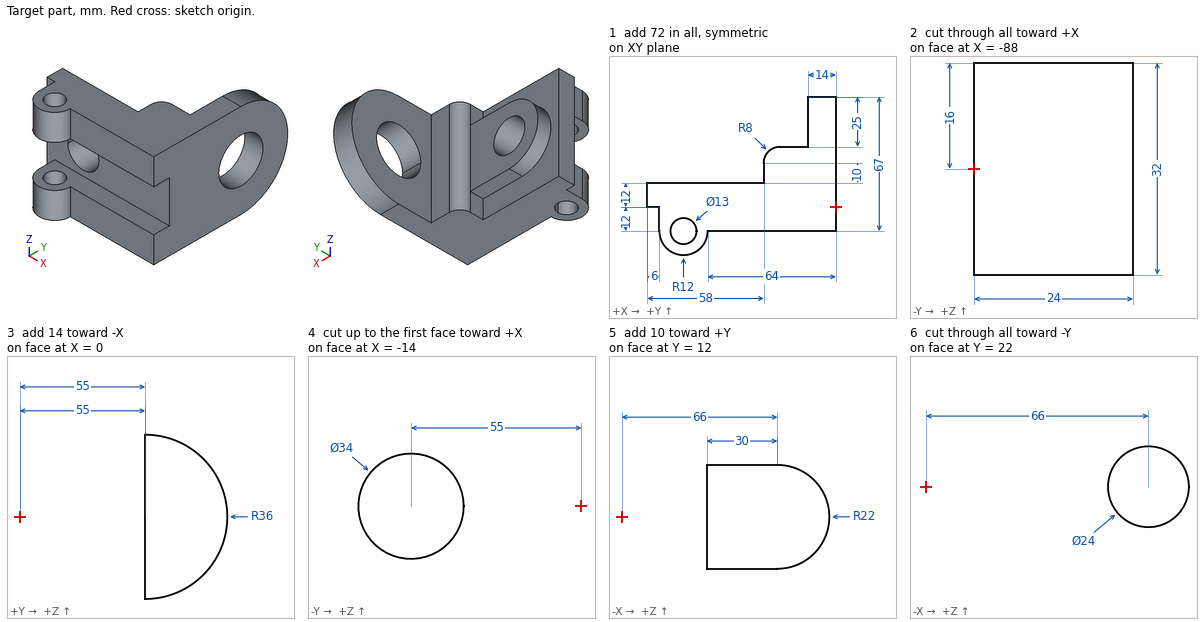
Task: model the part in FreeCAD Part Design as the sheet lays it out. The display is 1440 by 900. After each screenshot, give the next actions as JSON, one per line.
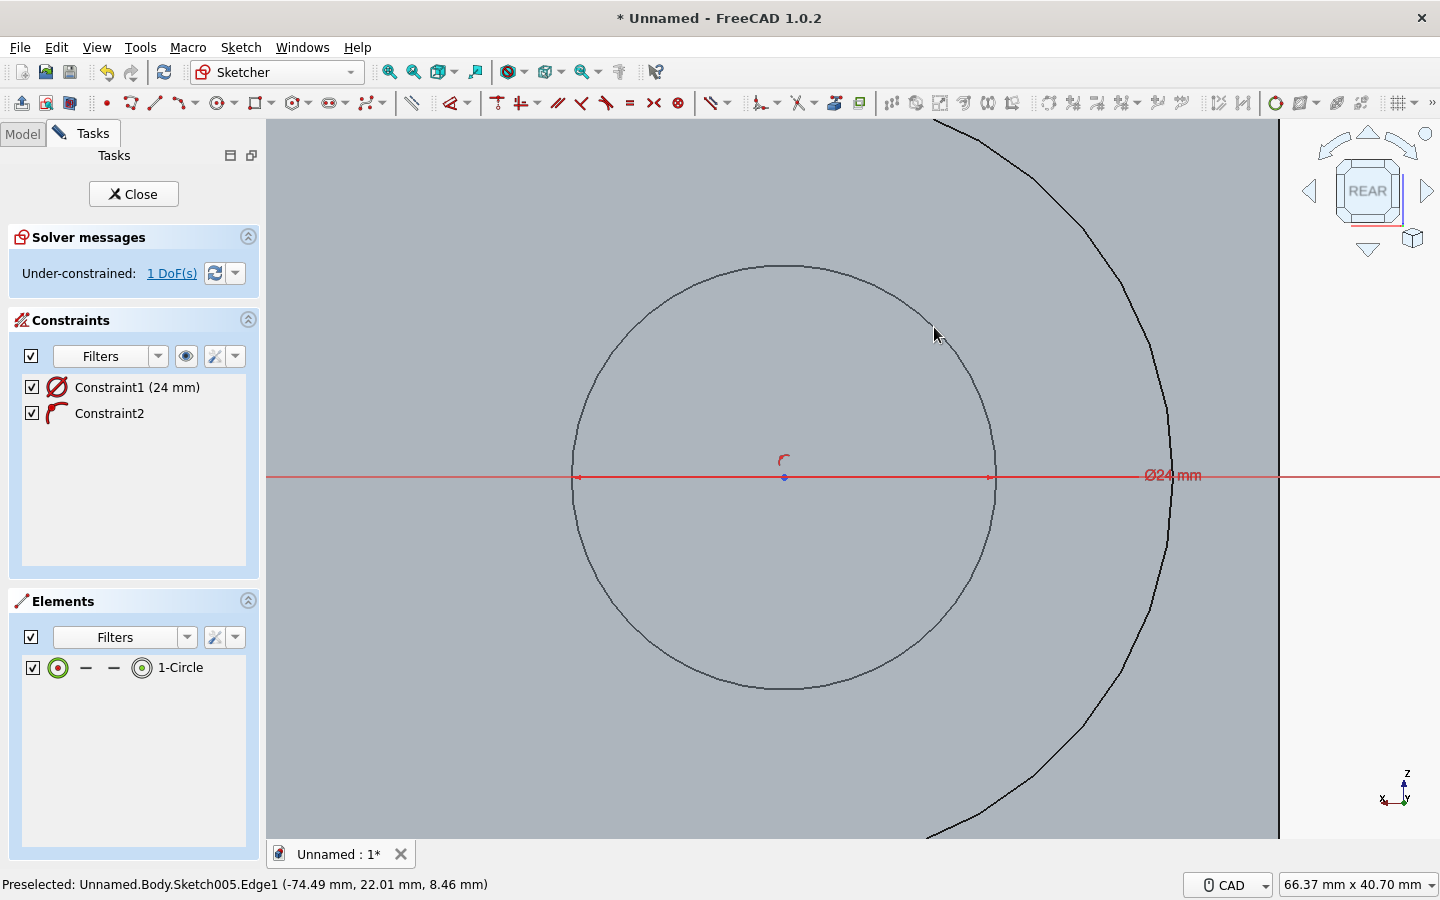
{"action": "left_click", "coordinate": [450, 104]}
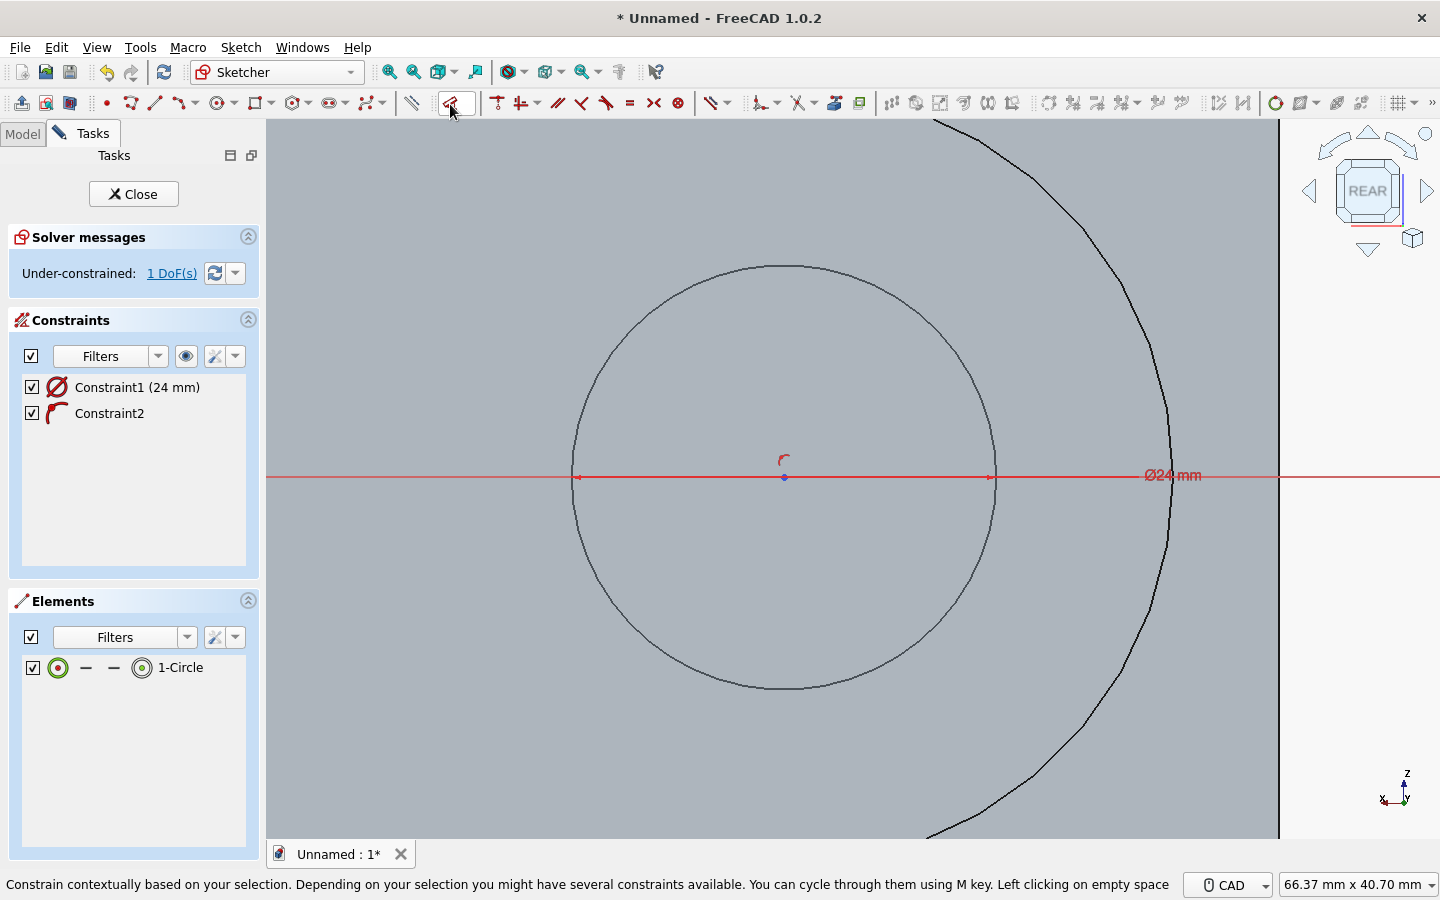
{"action": "left_click", "coordinate": [784, 477]}
{"action": "left_click", "coordinate": [539, 511]}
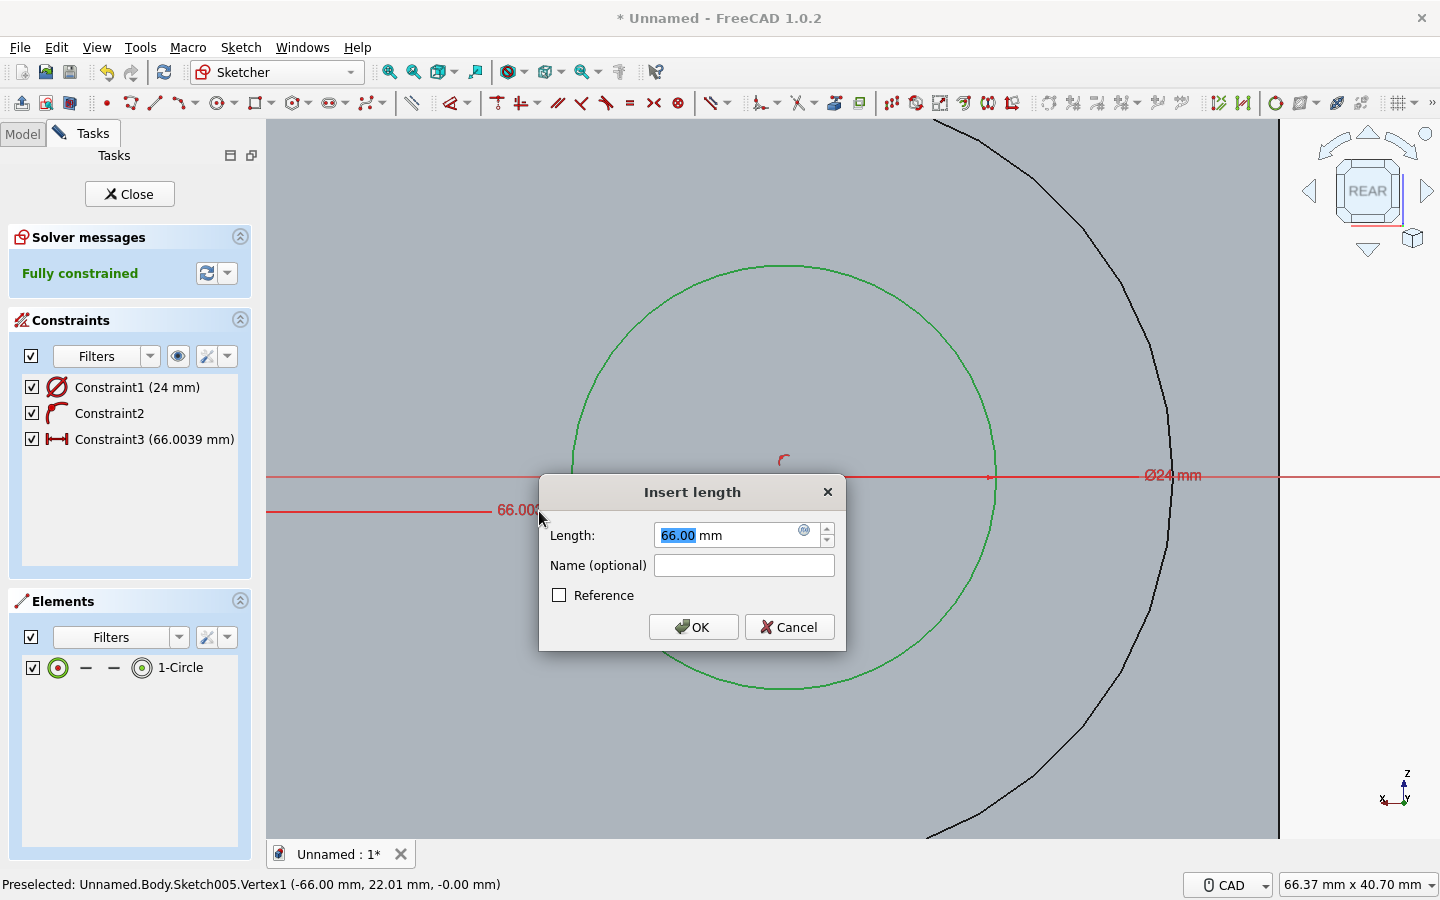
{"action": "type", "text": "66"}
{"action": "key", "text": "Return"}
{"action": "key", "text": "Escape"}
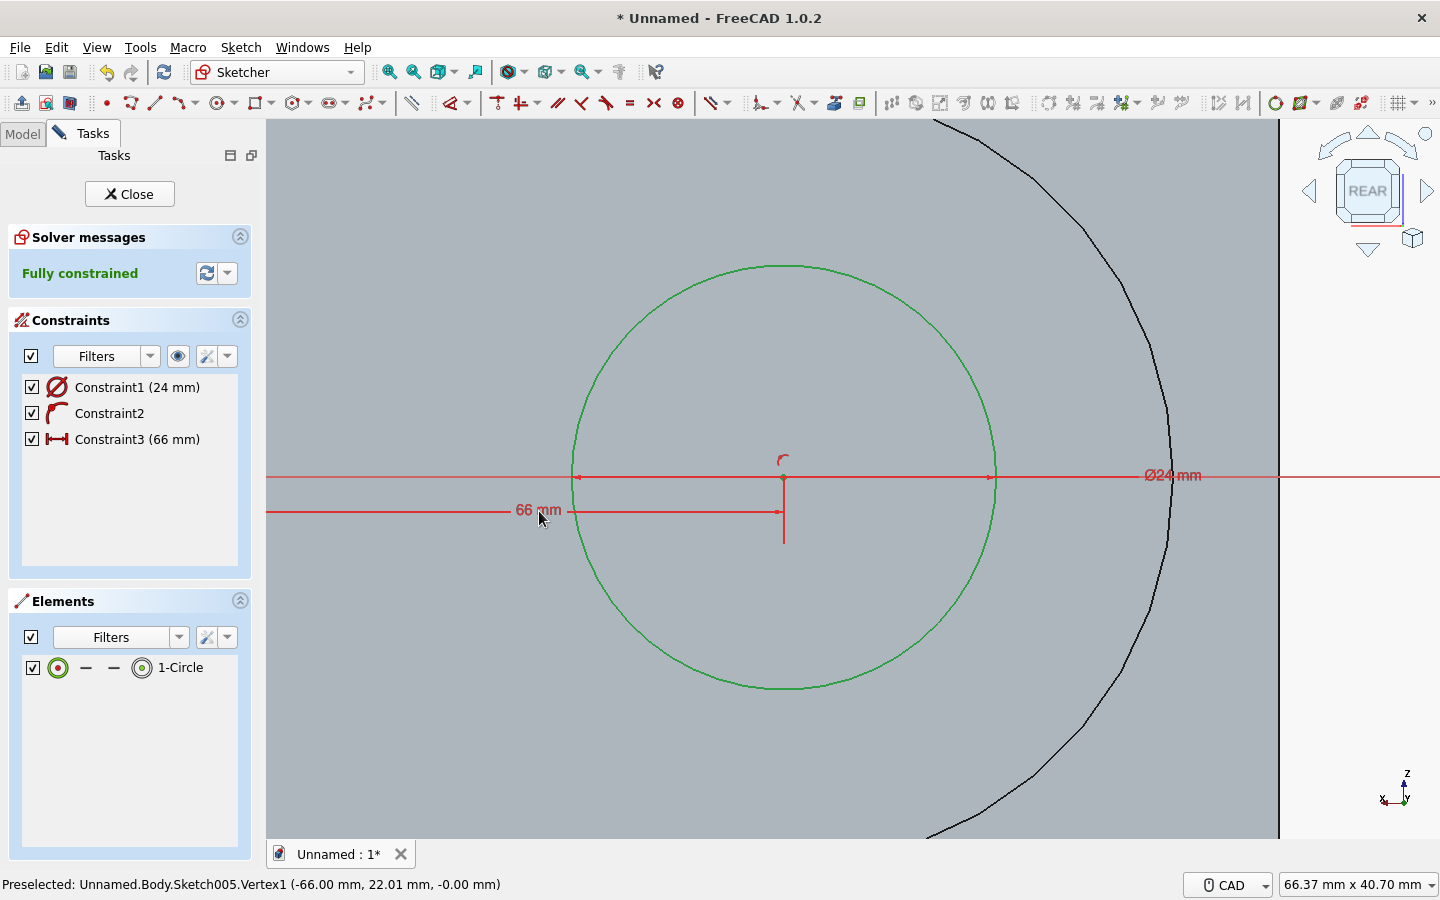
{"action": "left_click", "coordinate": [130, 194]}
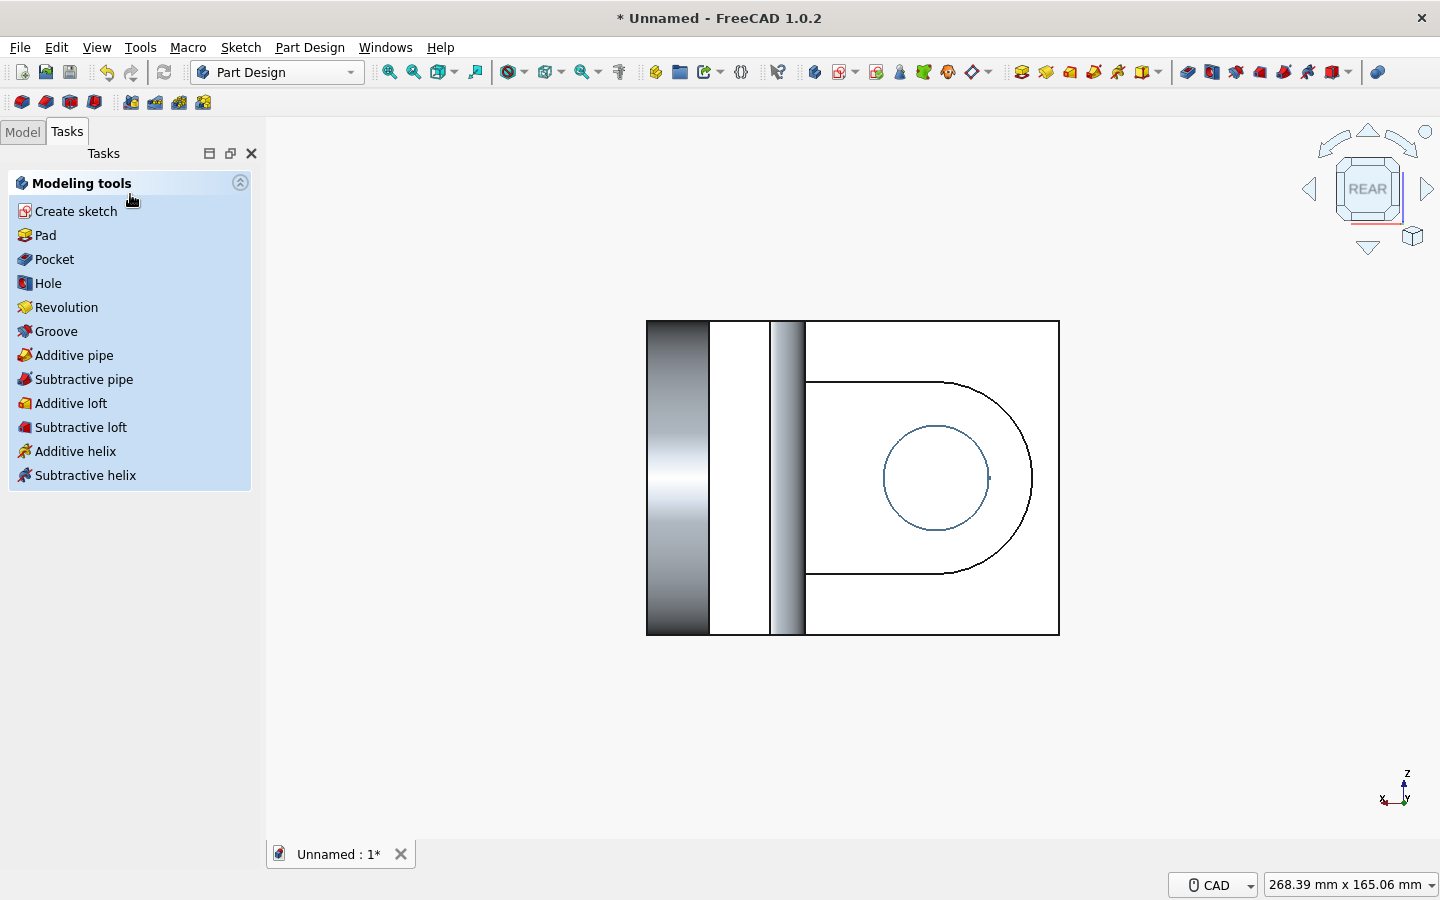
{"action": "left_click", "coordinate": [1188, 72]}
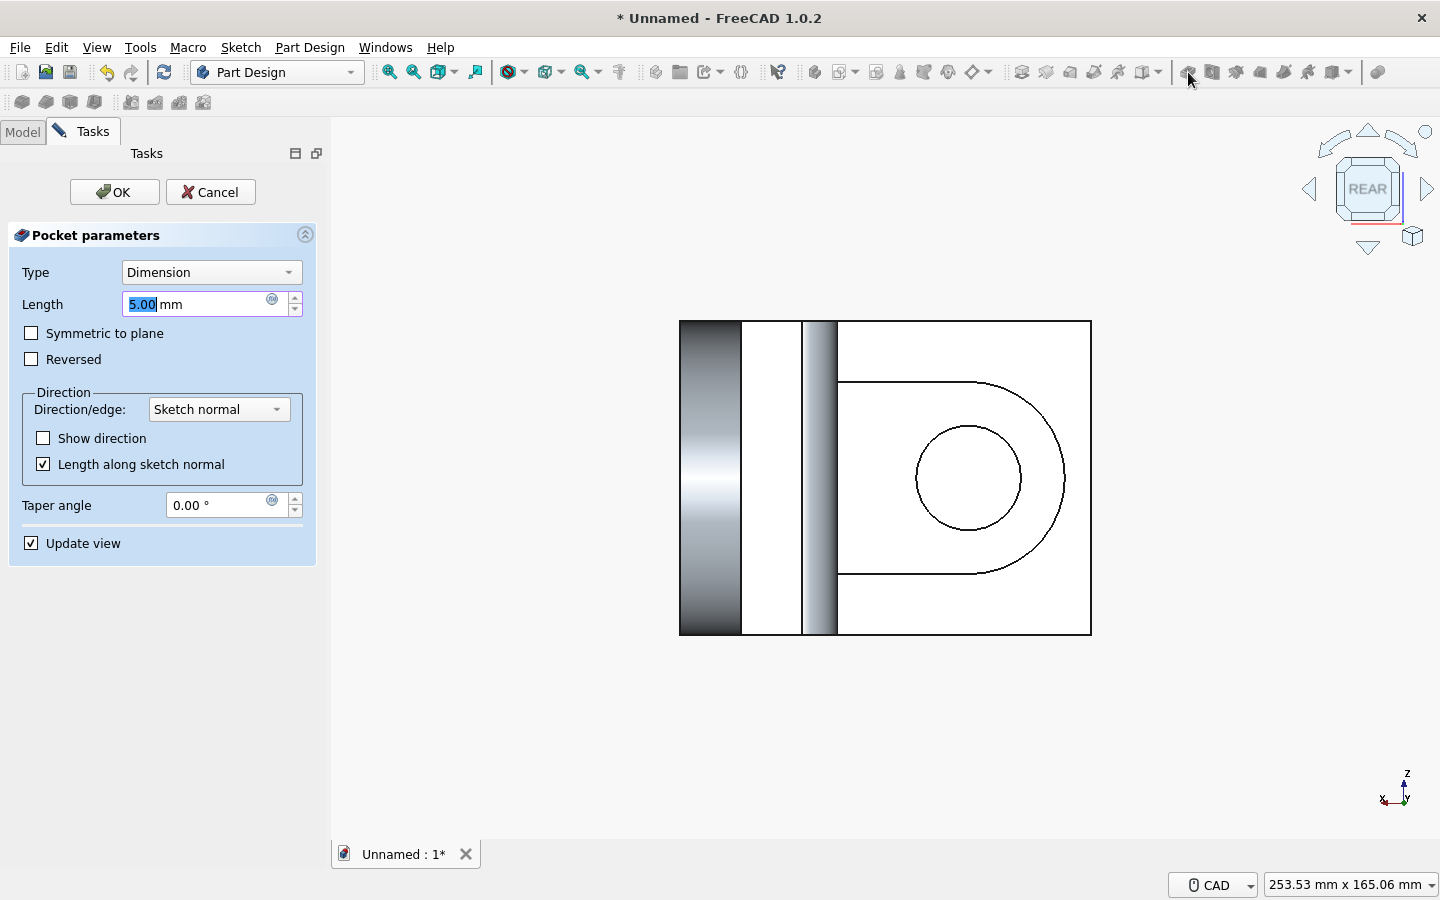
{"action": "left_click", "coordinate": [212, 272]}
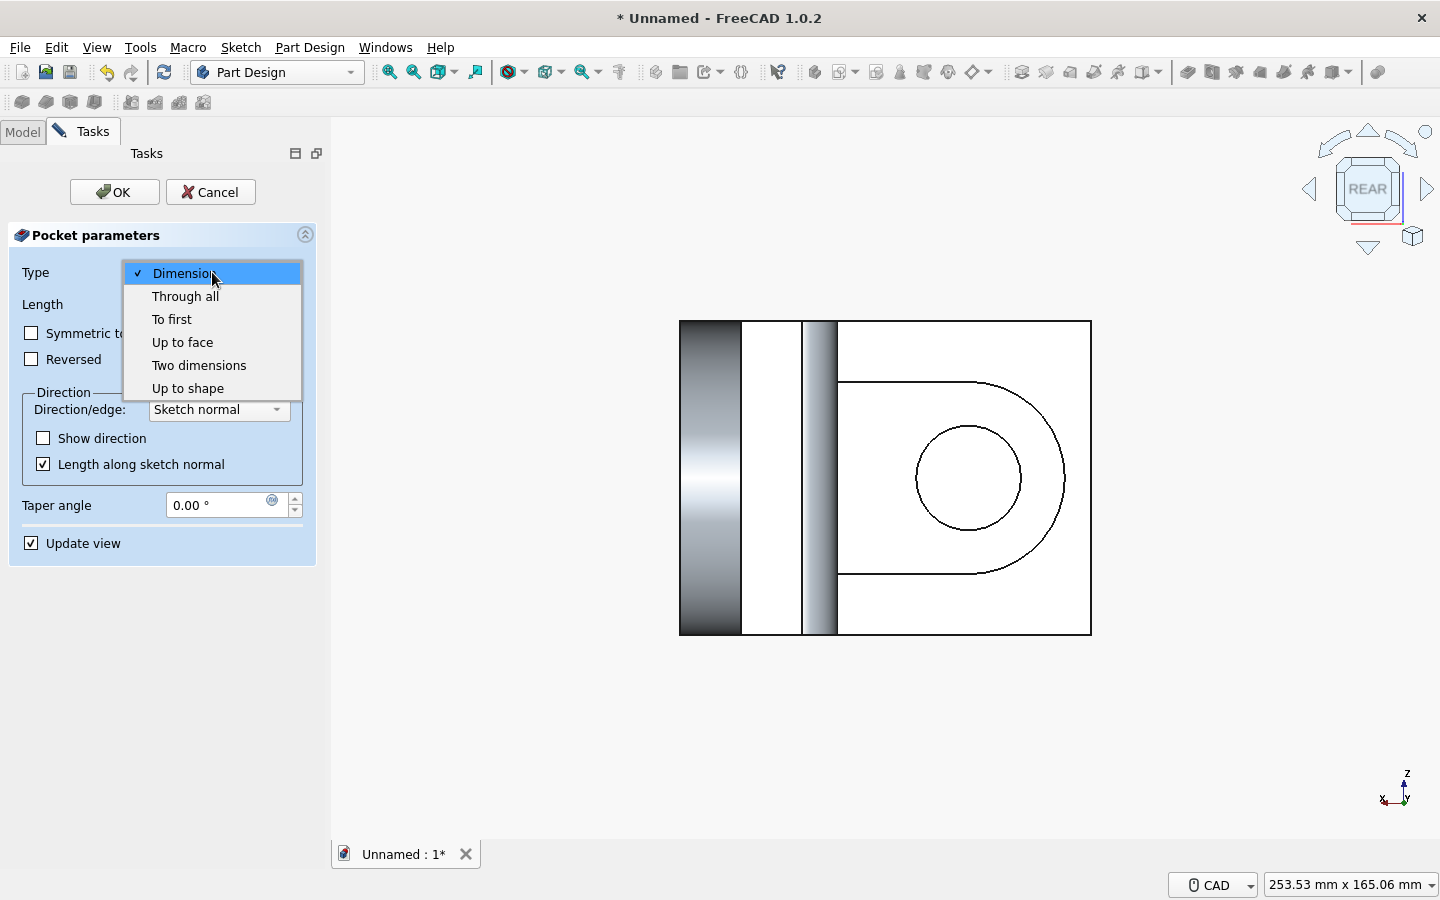
{"action": "left_click", "coordinate": [212, 296]}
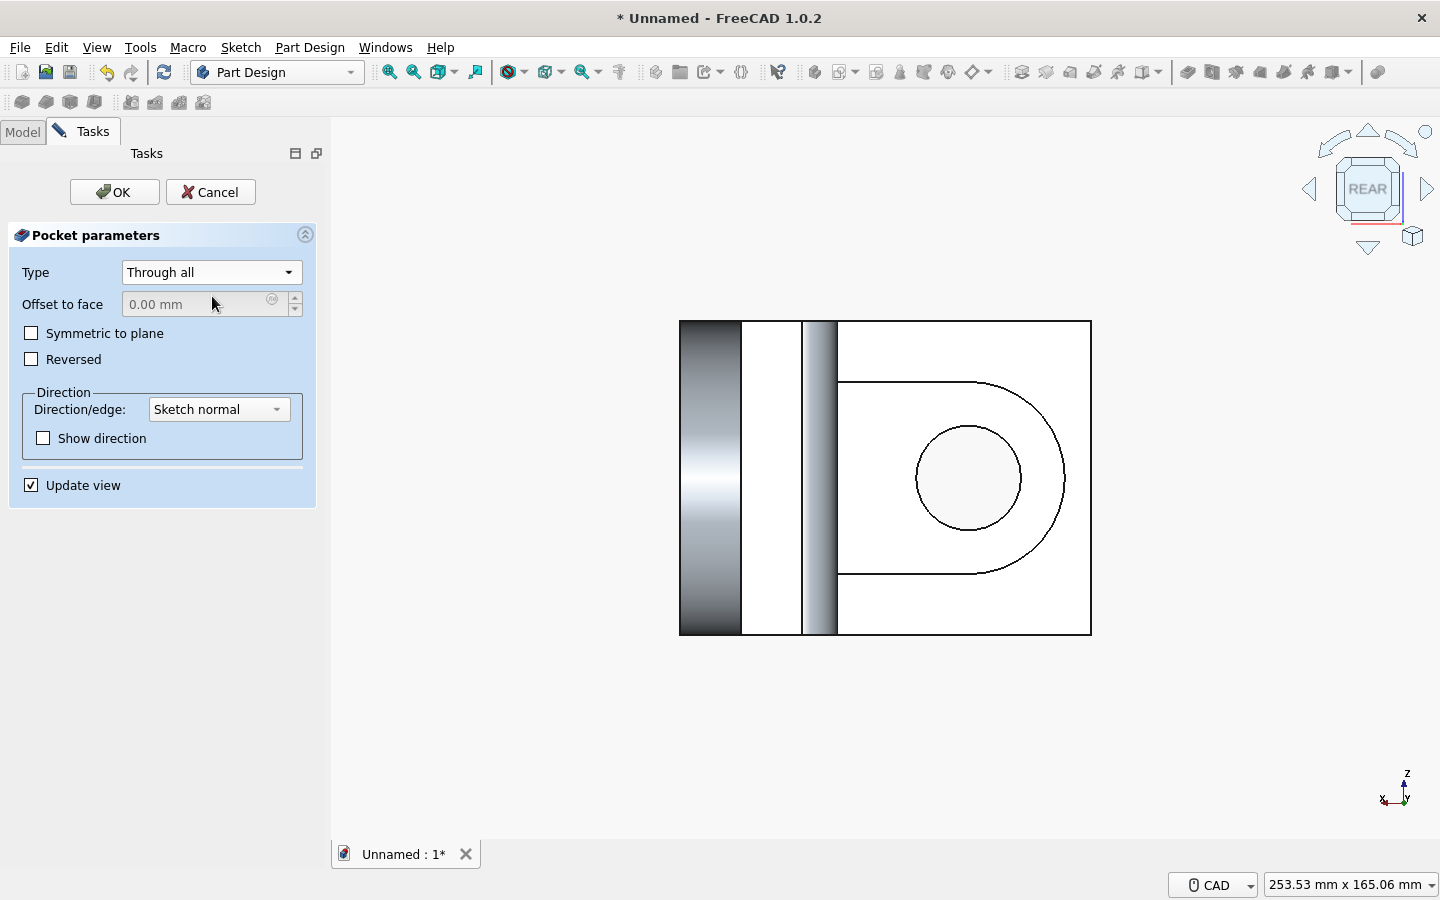
{"action": "left_click", "coordinate": [115, 192]}